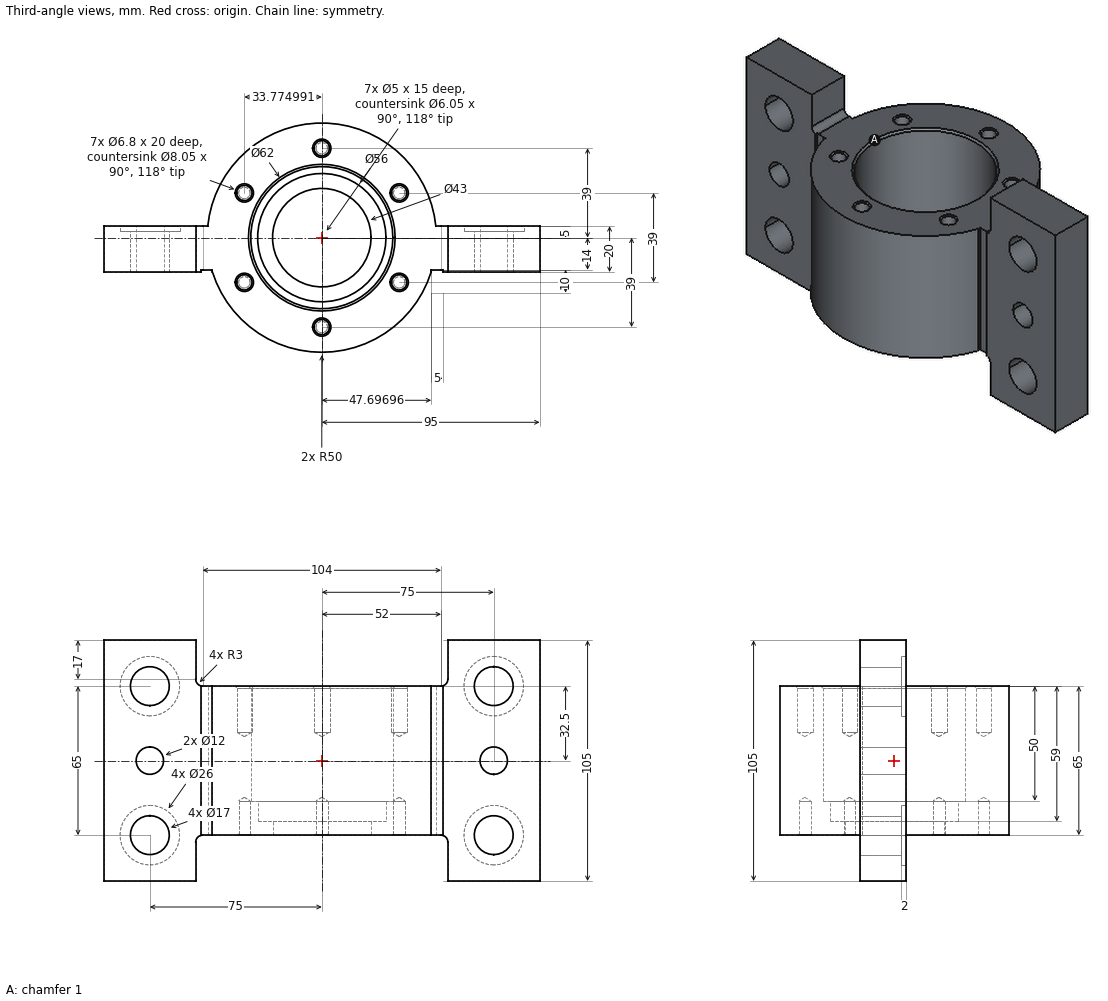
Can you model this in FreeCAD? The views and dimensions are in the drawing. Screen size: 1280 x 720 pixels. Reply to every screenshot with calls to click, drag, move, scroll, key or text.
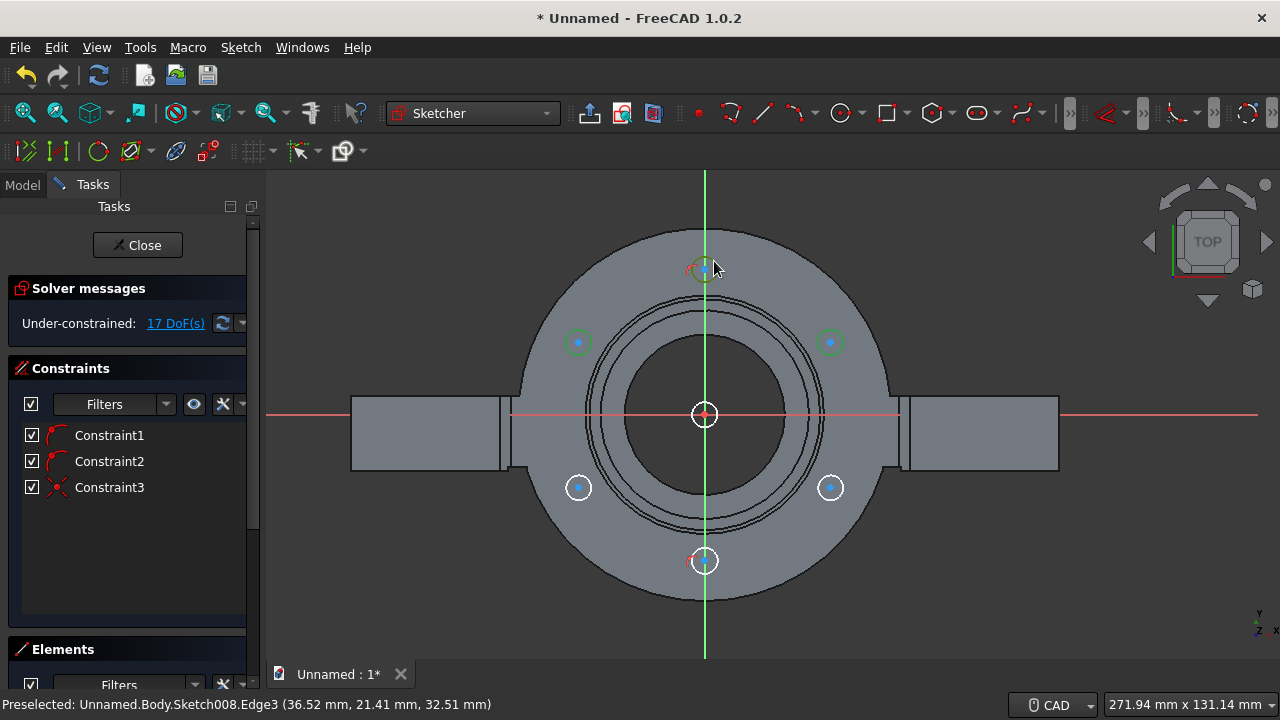
click(839, 479)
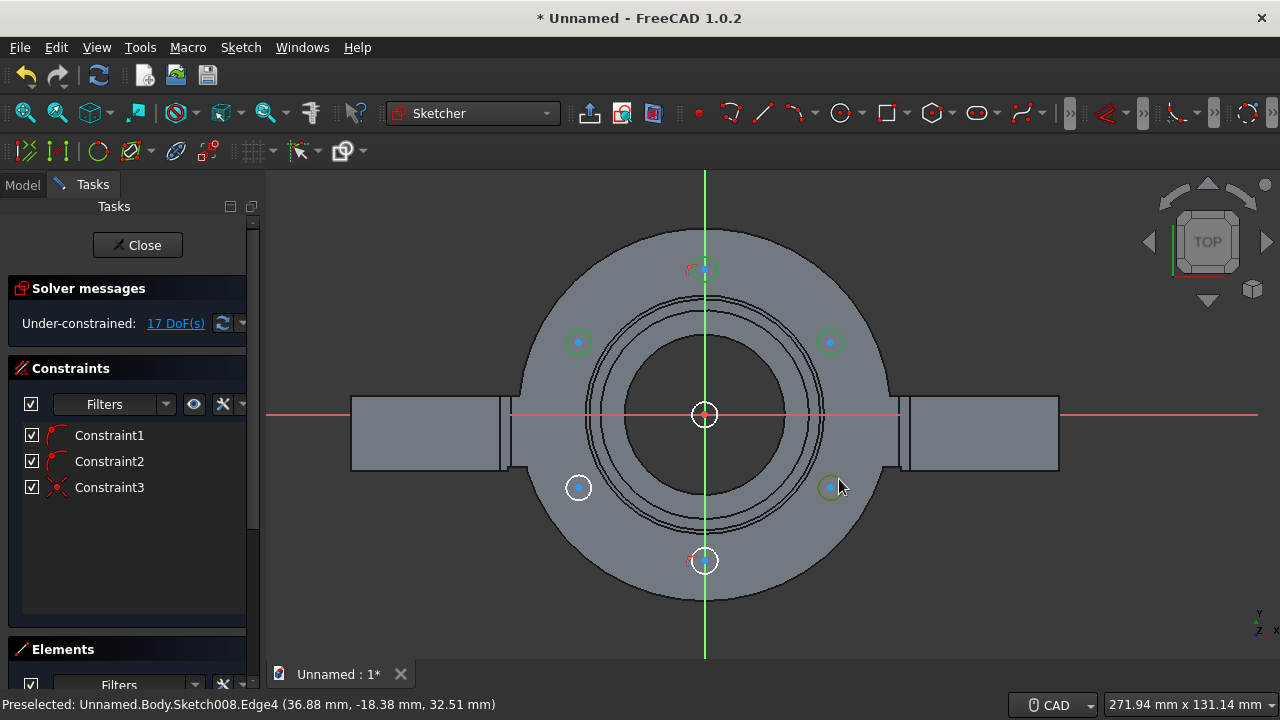
scroll(714, 552, up, 3)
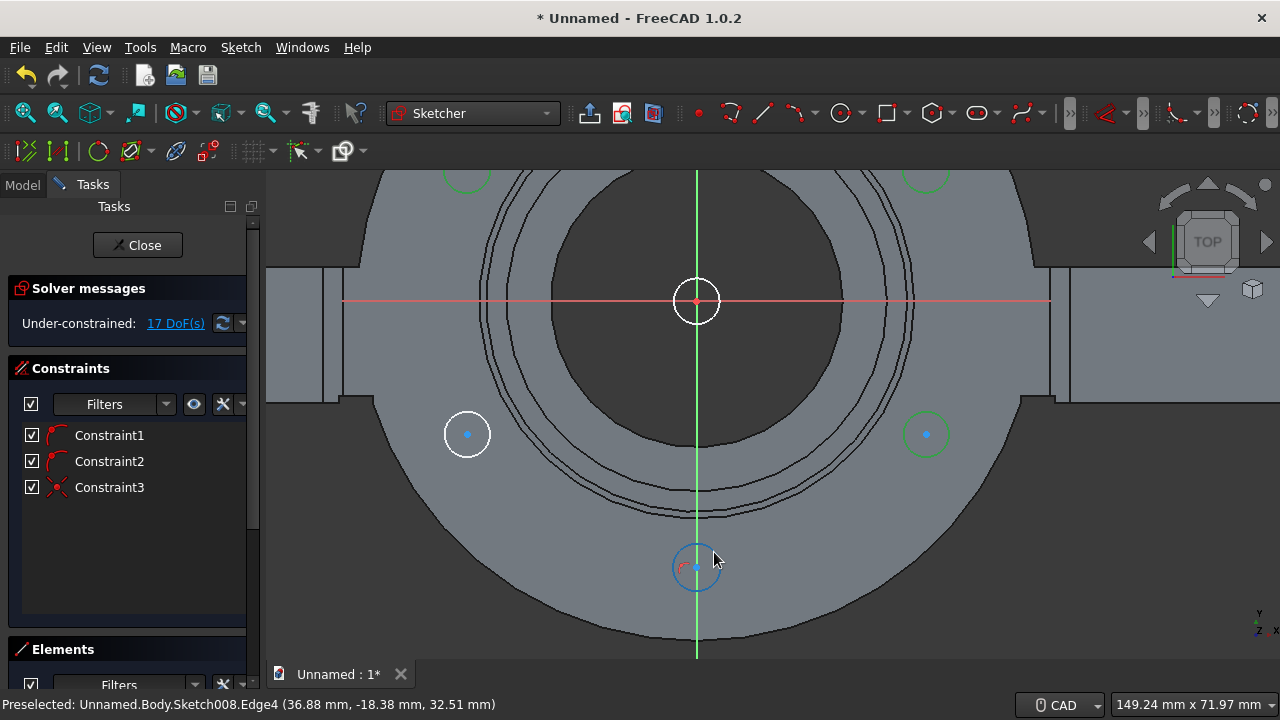
click(713, 551)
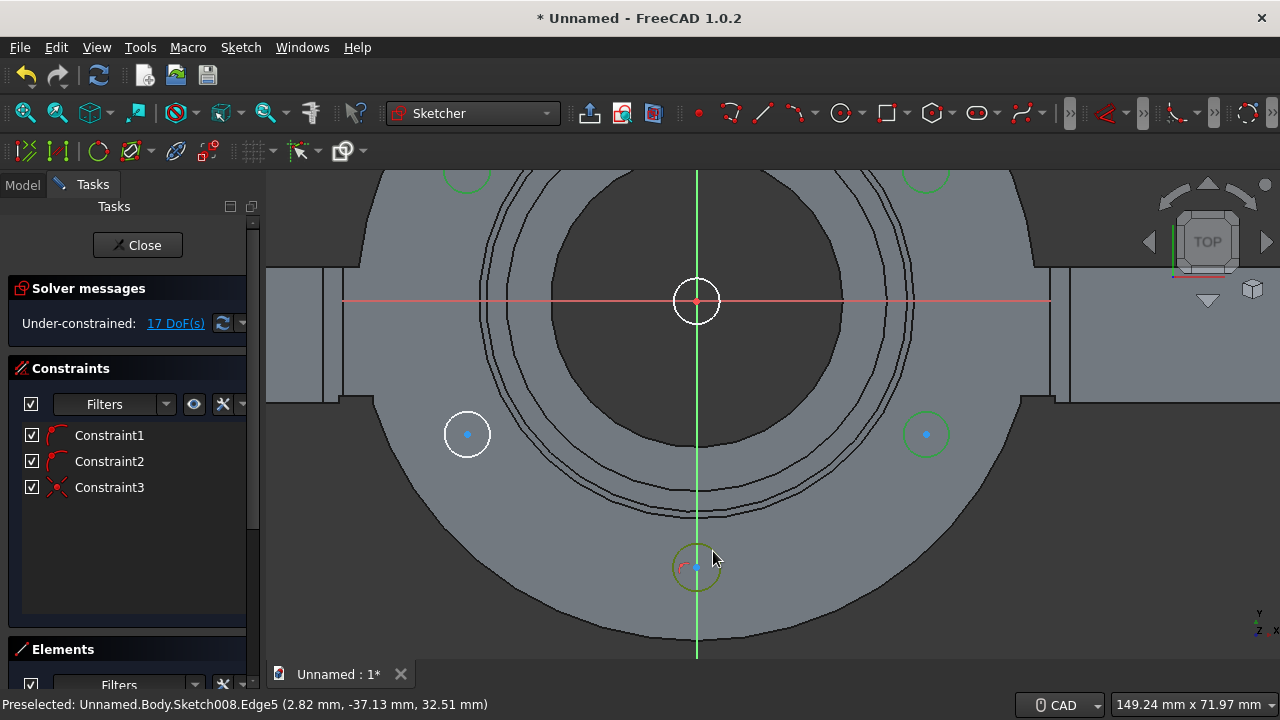
click(483, 418)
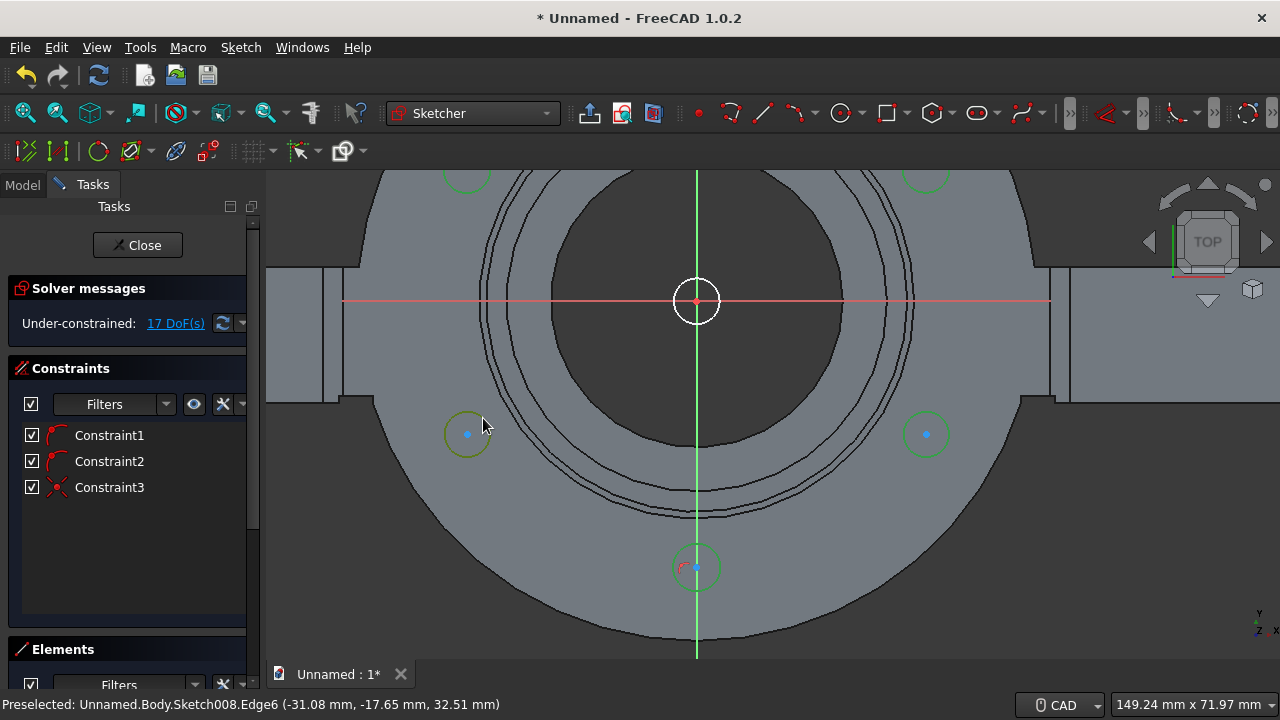
click(713, 285)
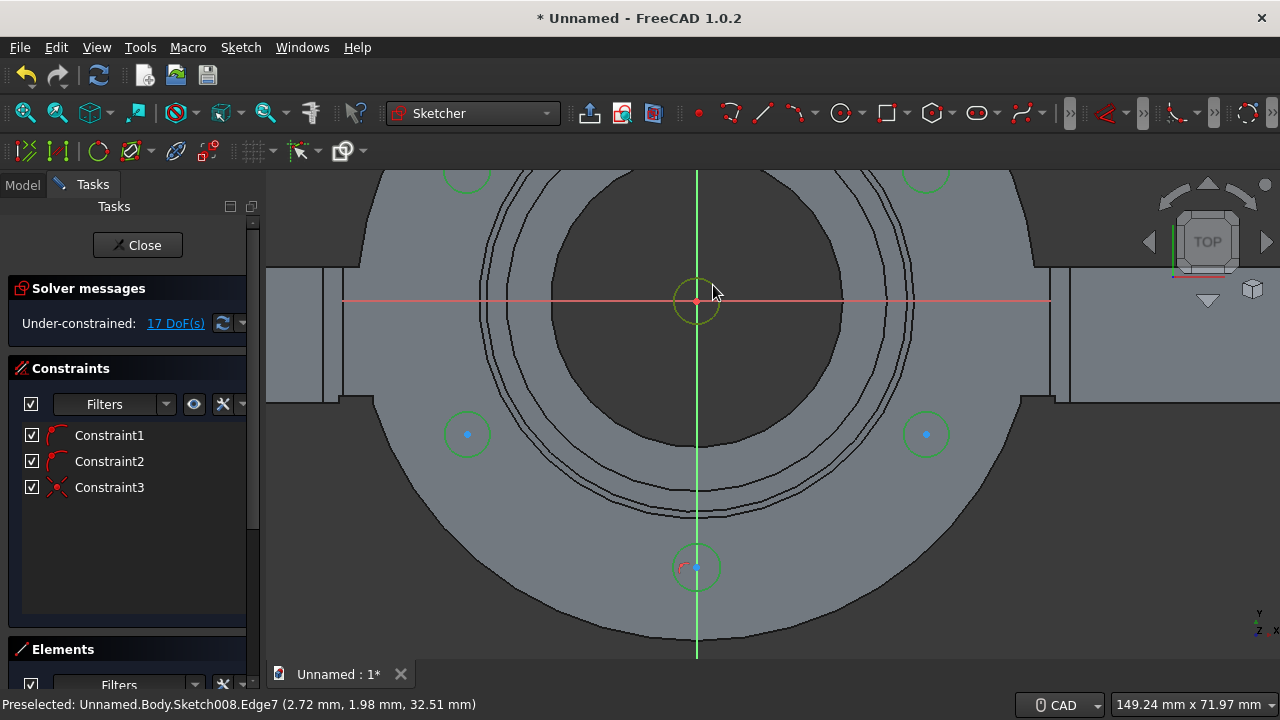
key(e)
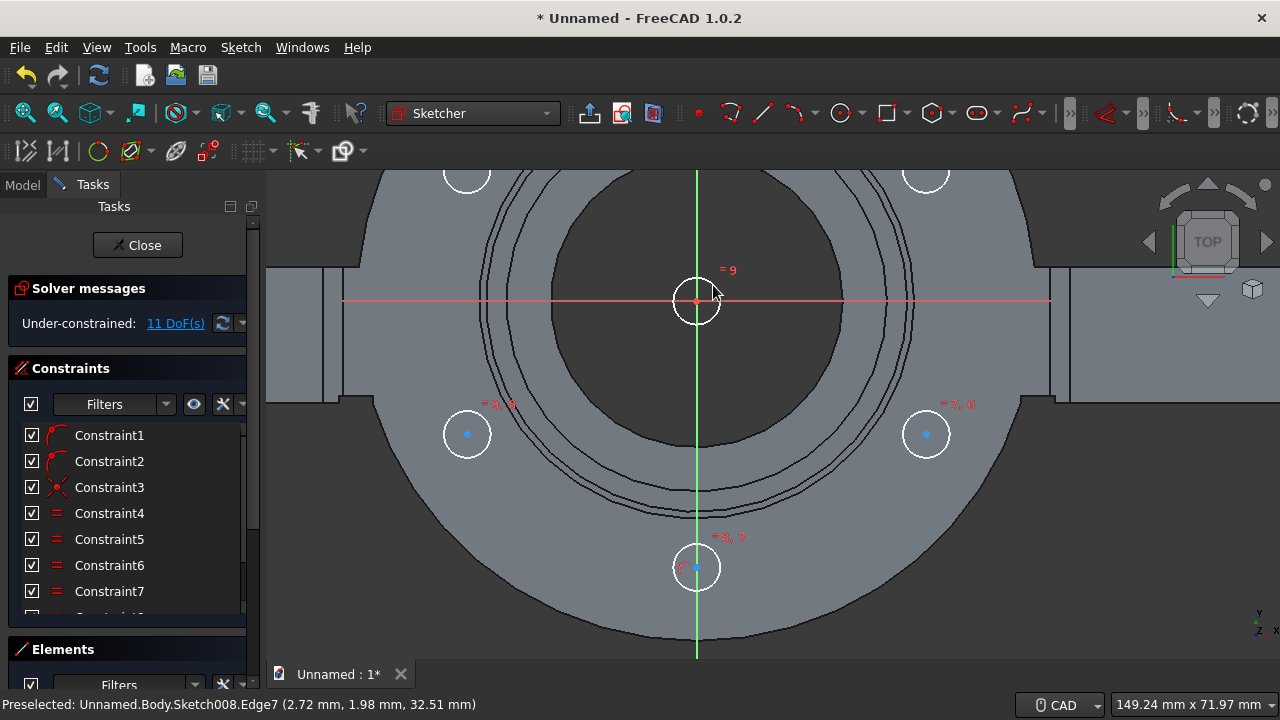
scroll(714, 552, down, 3)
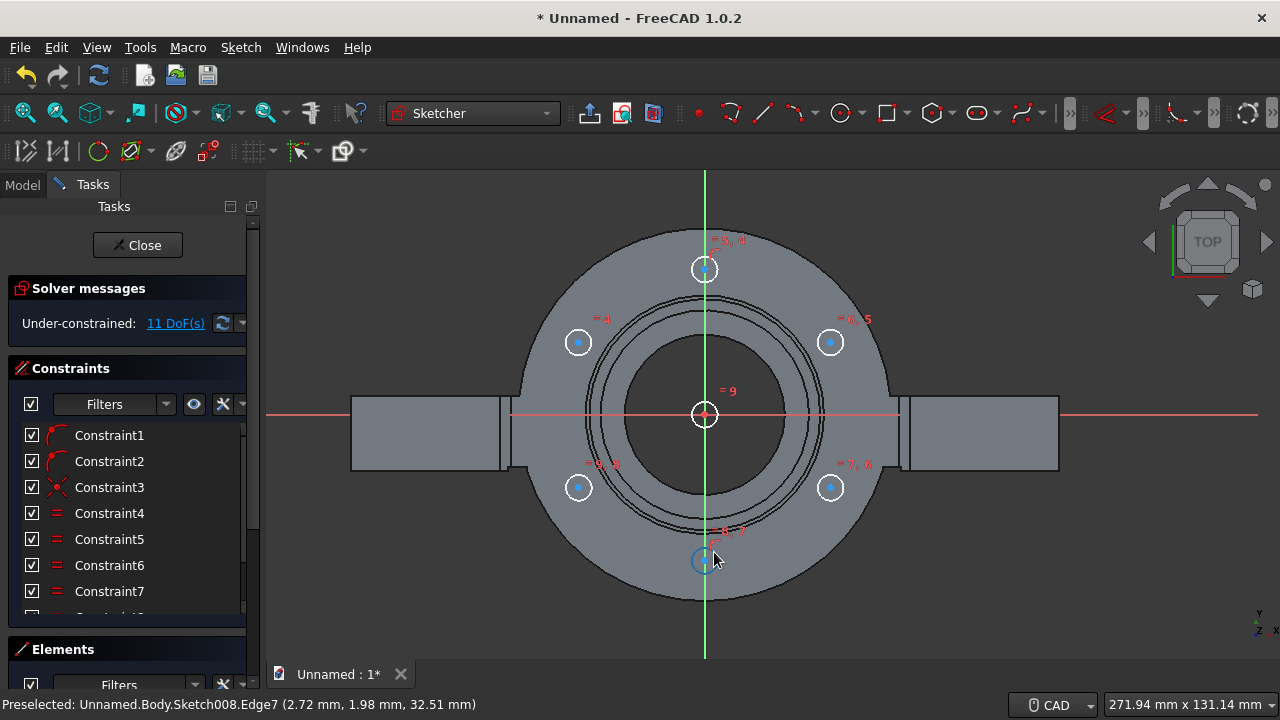
click(579, 343)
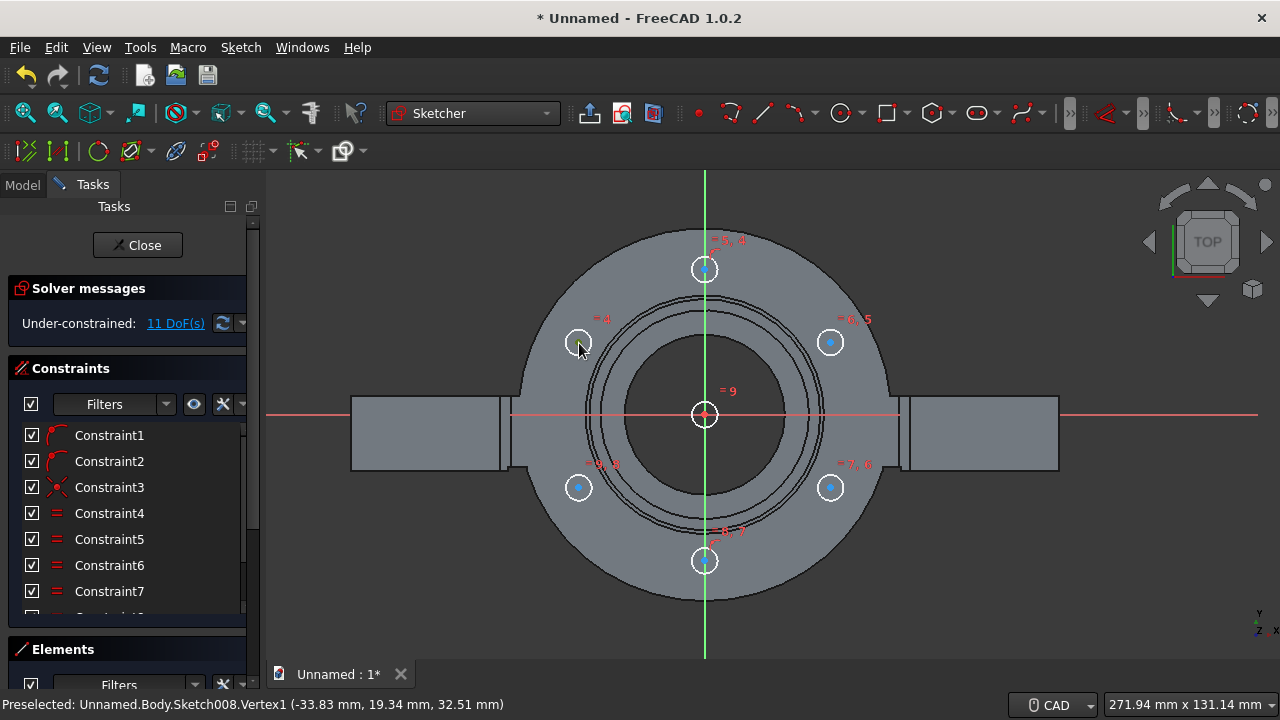
click(831, 342)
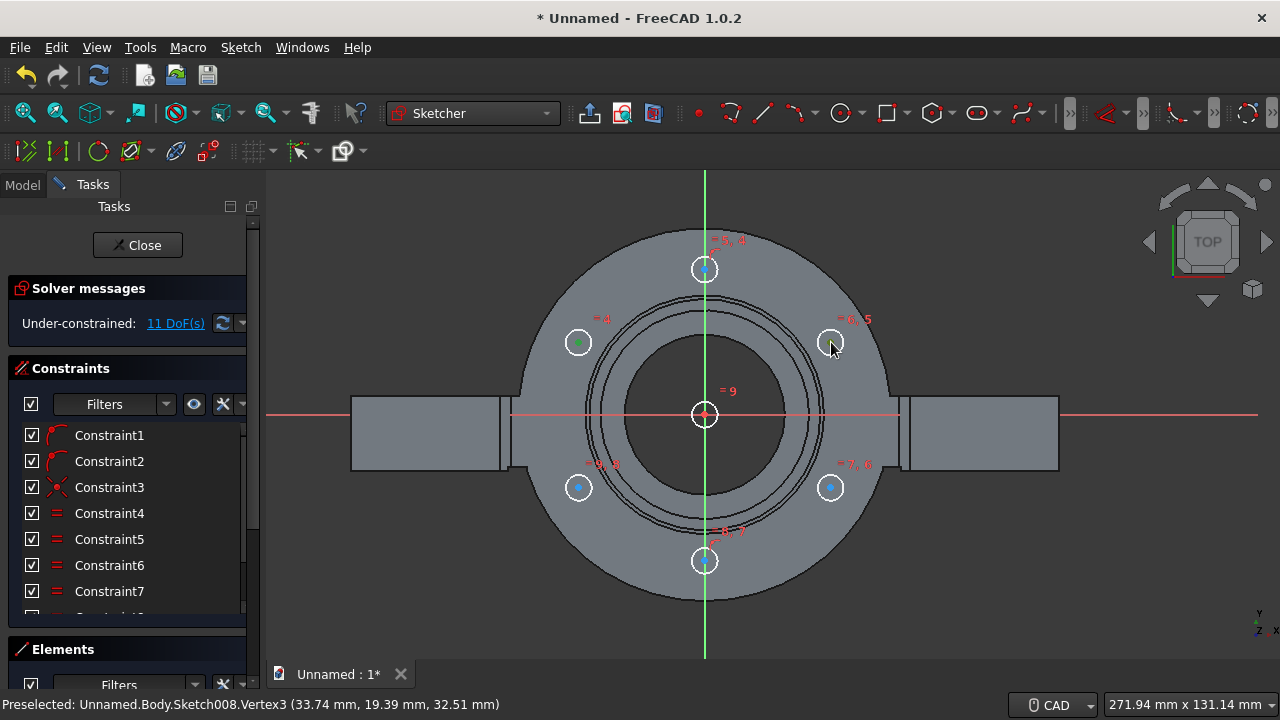
click(705, 507)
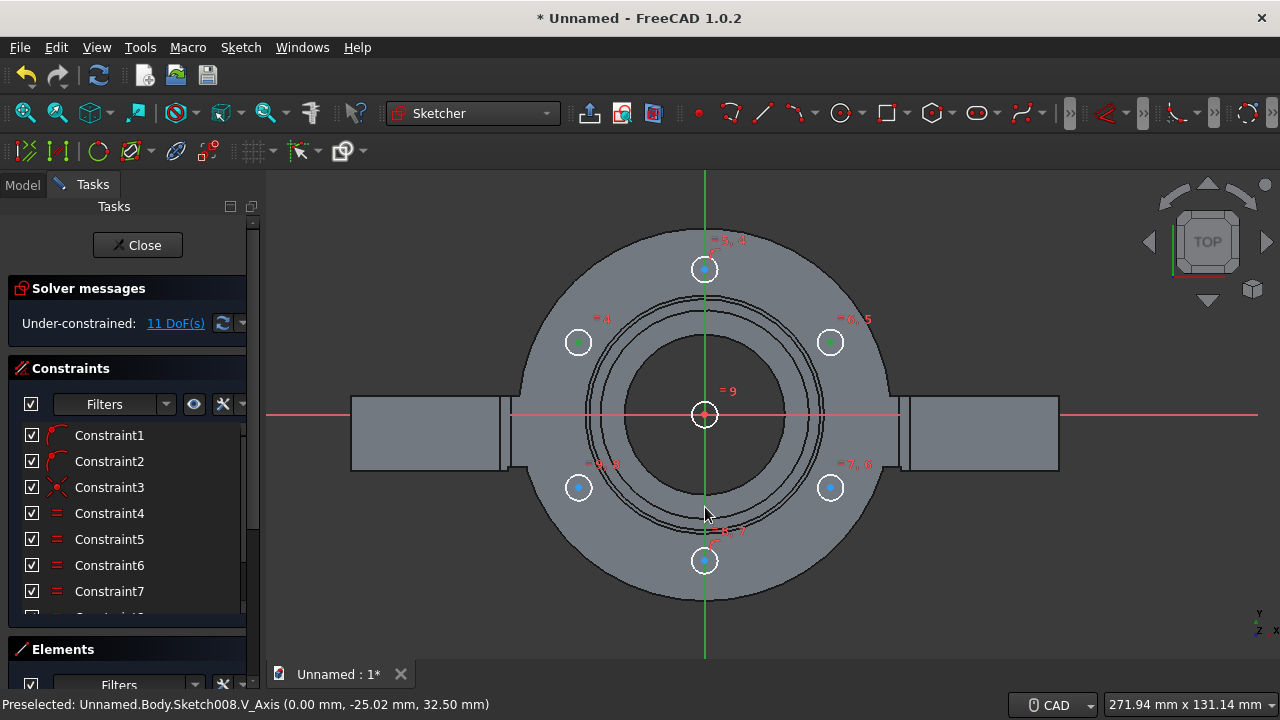
key(s)